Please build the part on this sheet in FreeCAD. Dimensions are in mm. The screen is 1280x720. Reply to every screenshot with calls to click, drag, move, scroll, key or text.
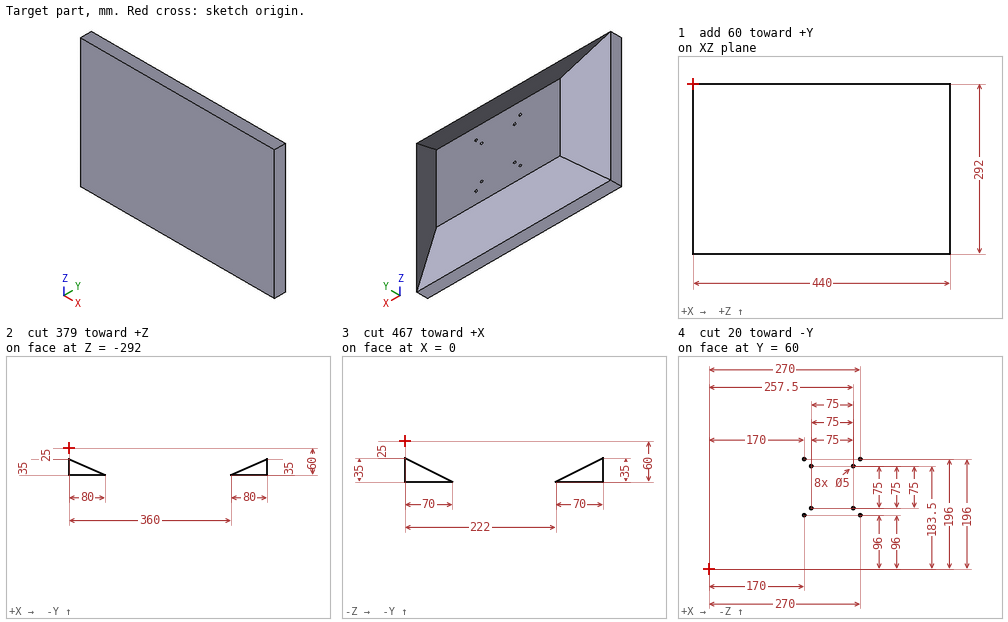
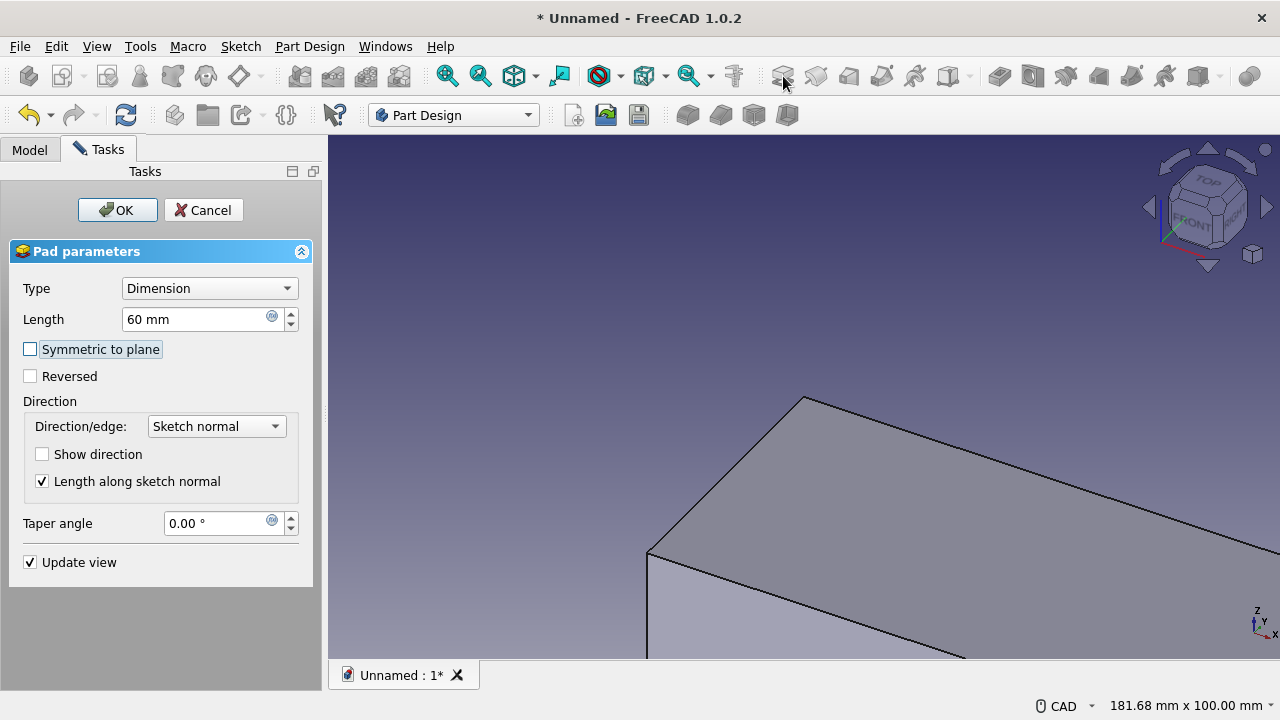
click(31, 376)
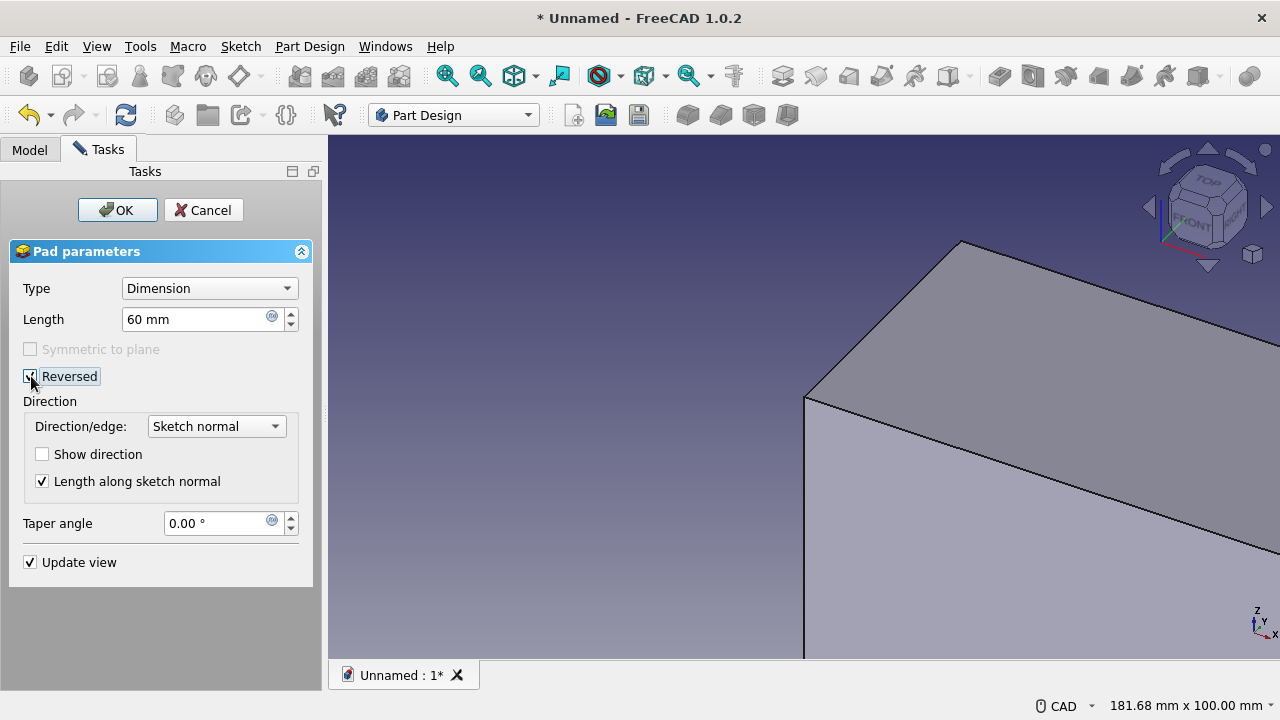
click(118, 210)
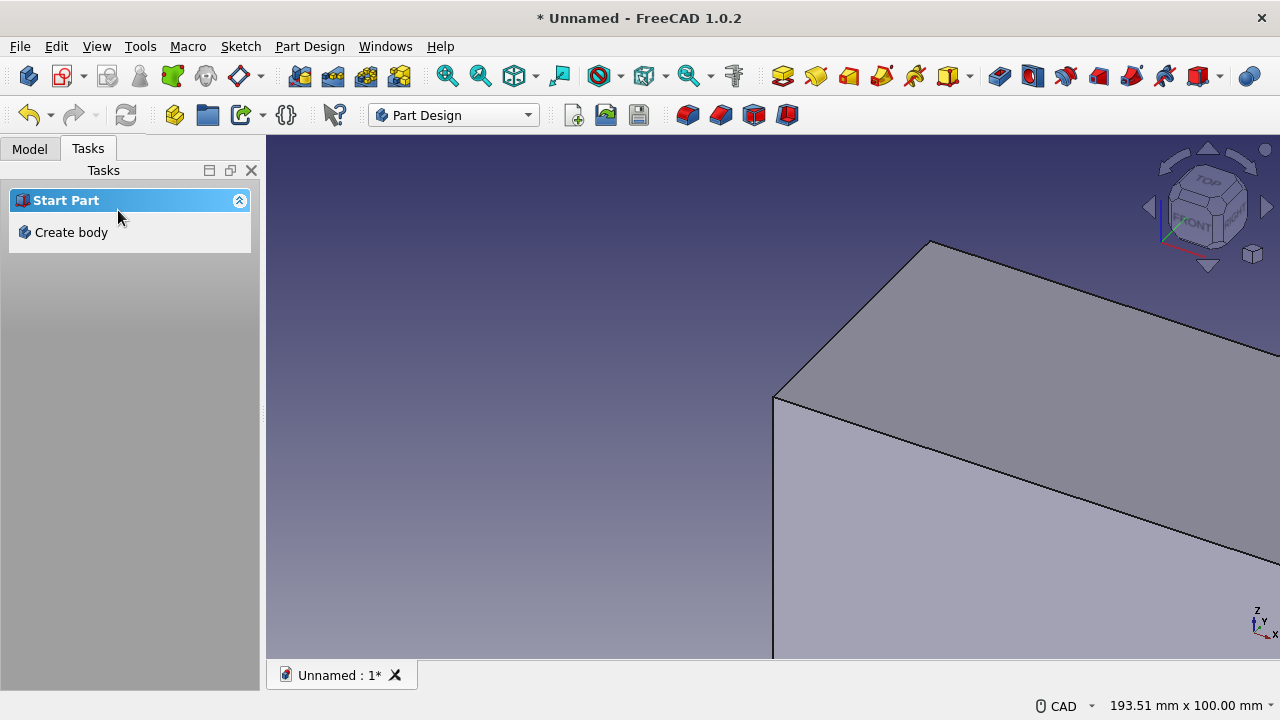
click(448, 76)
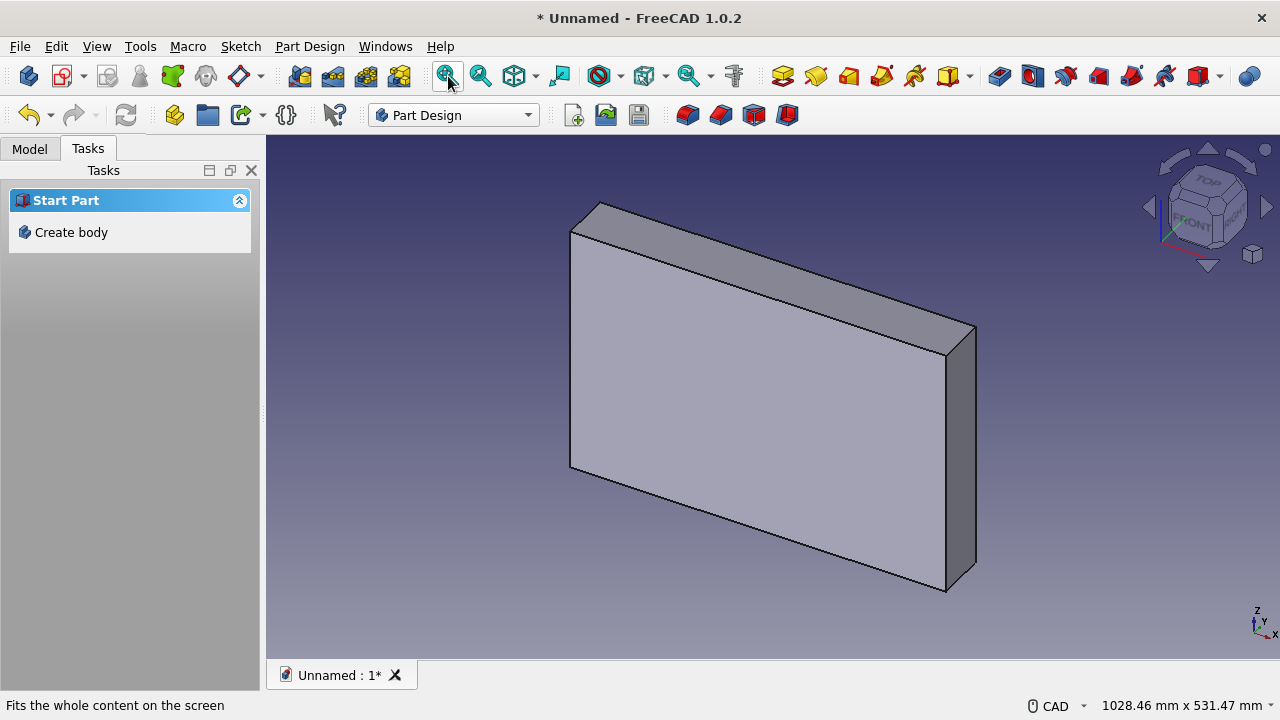
key(5)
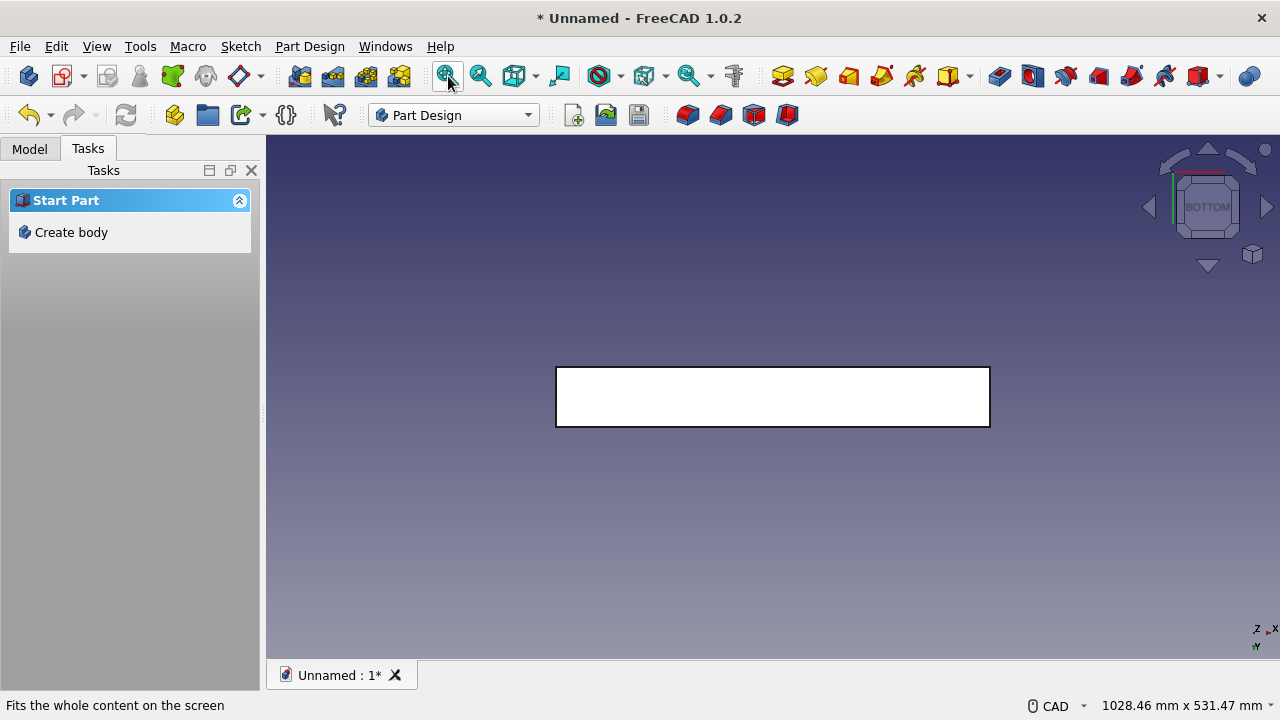
key(v)
key(f)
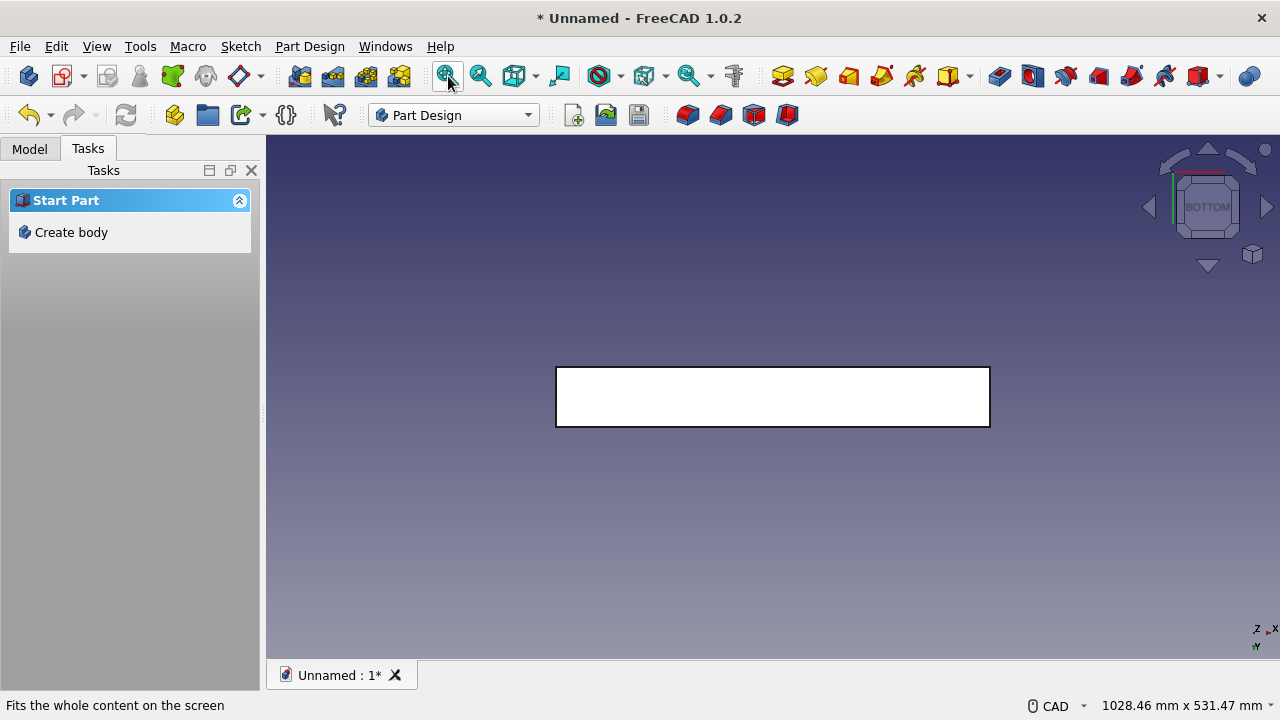
click(959, 396)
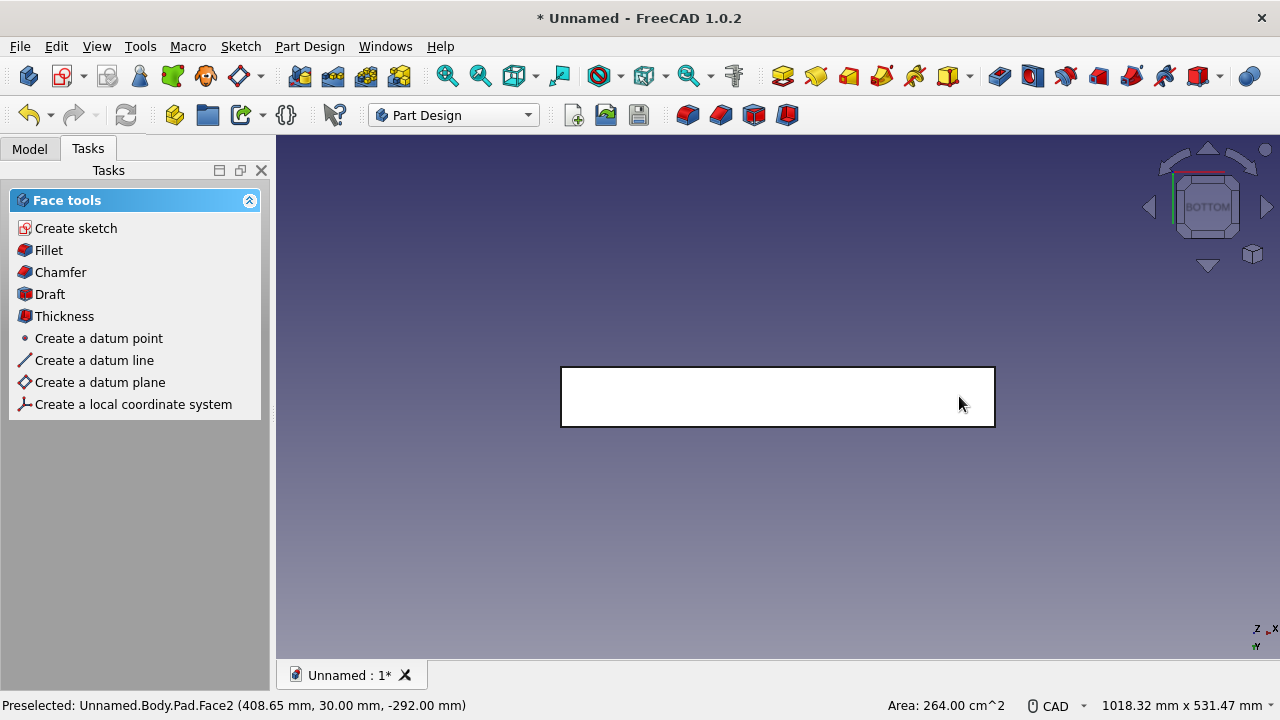
click(62, 76)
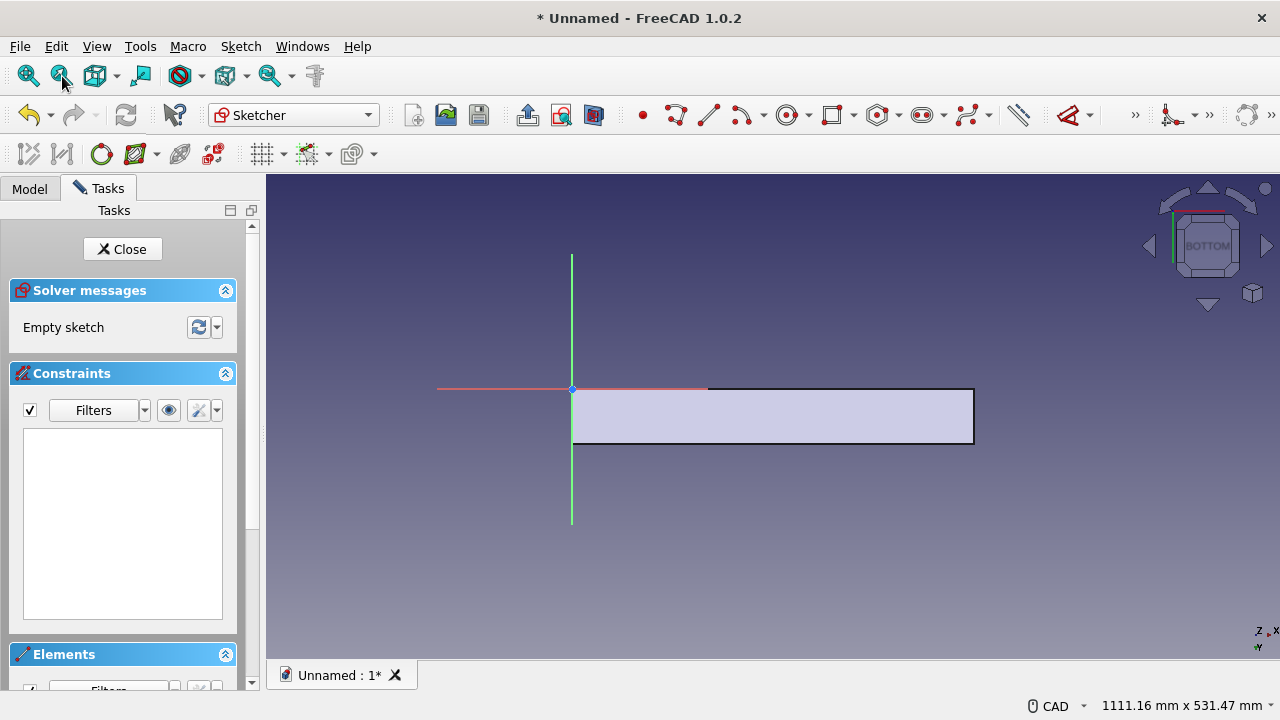
scroll(912, 416, up, 2)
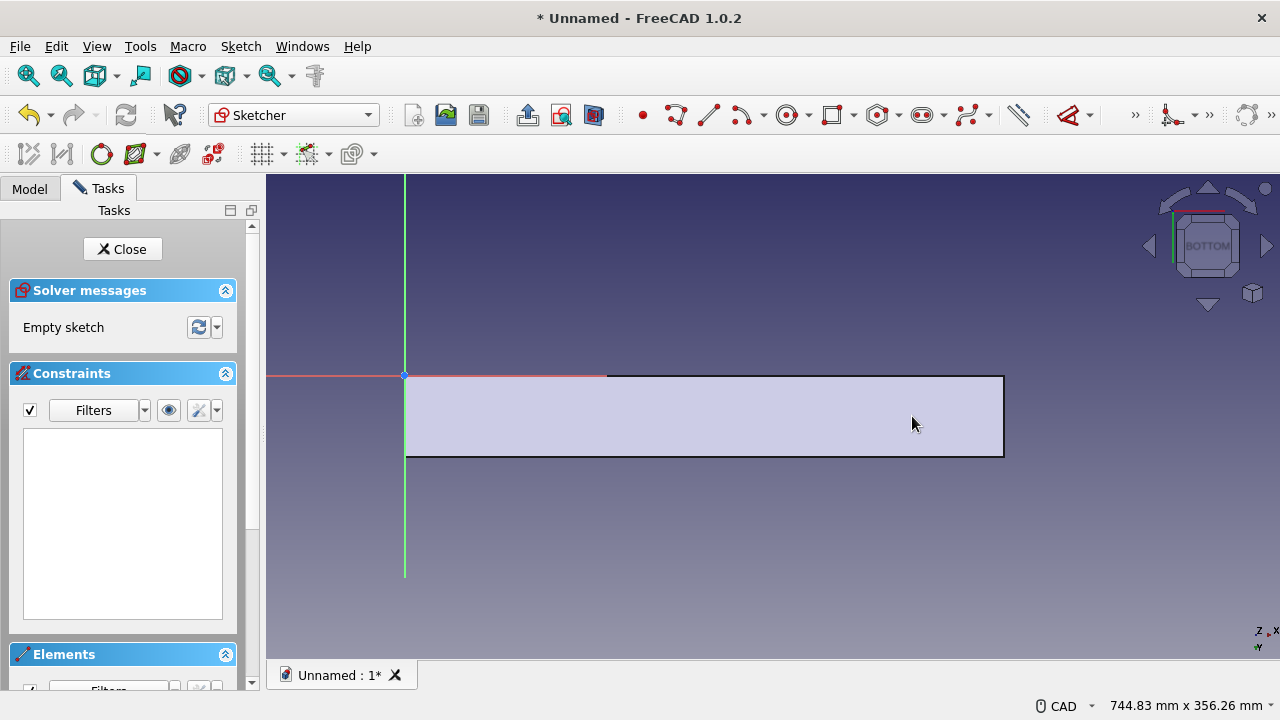
key(g)
key(m)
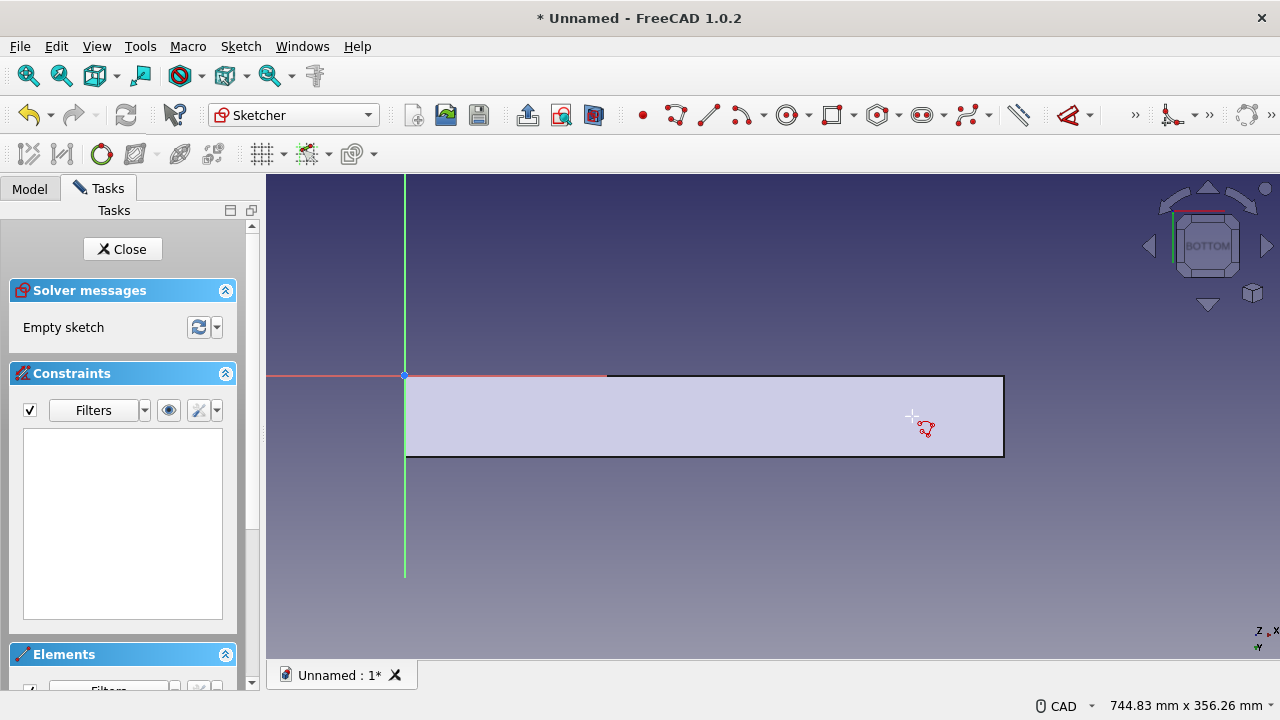
click(895, 457)
click(1004, 457)
click(1004, 410)
click(895, 458)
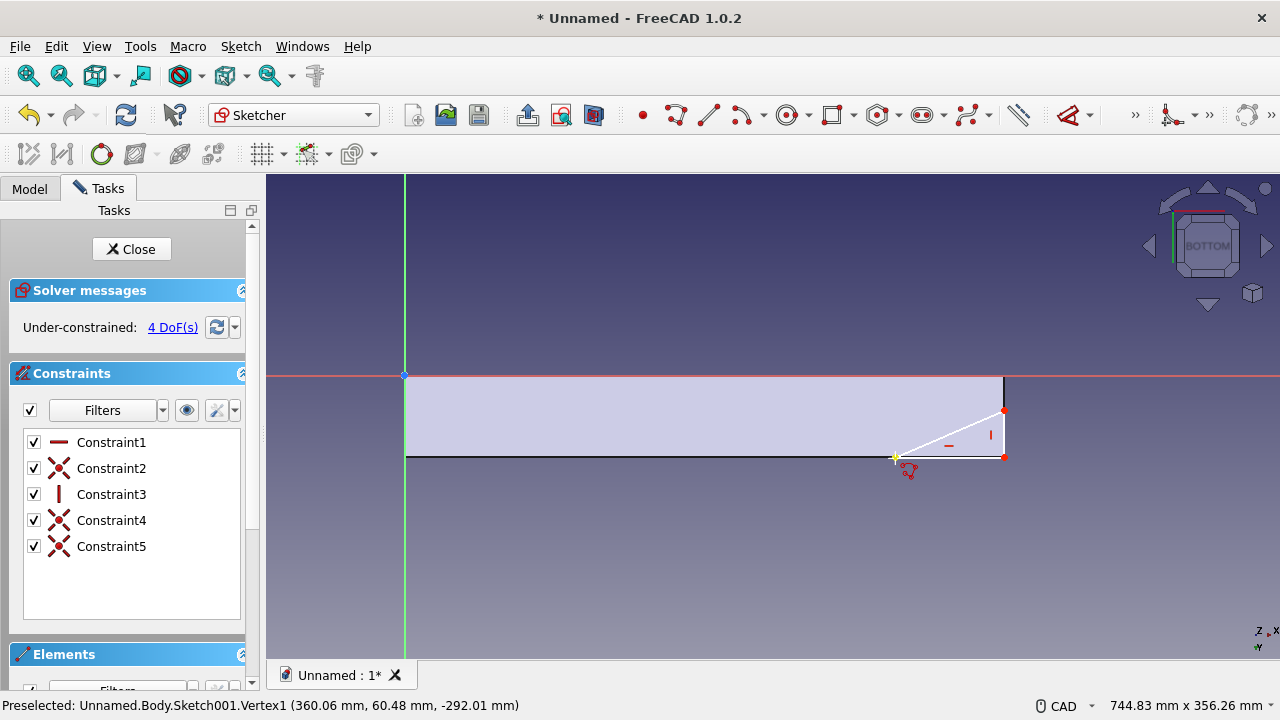
click(405, 410)
click(414, 457)
click(514, 457)
click(405, 411)
key(Escape)
key(Escape)